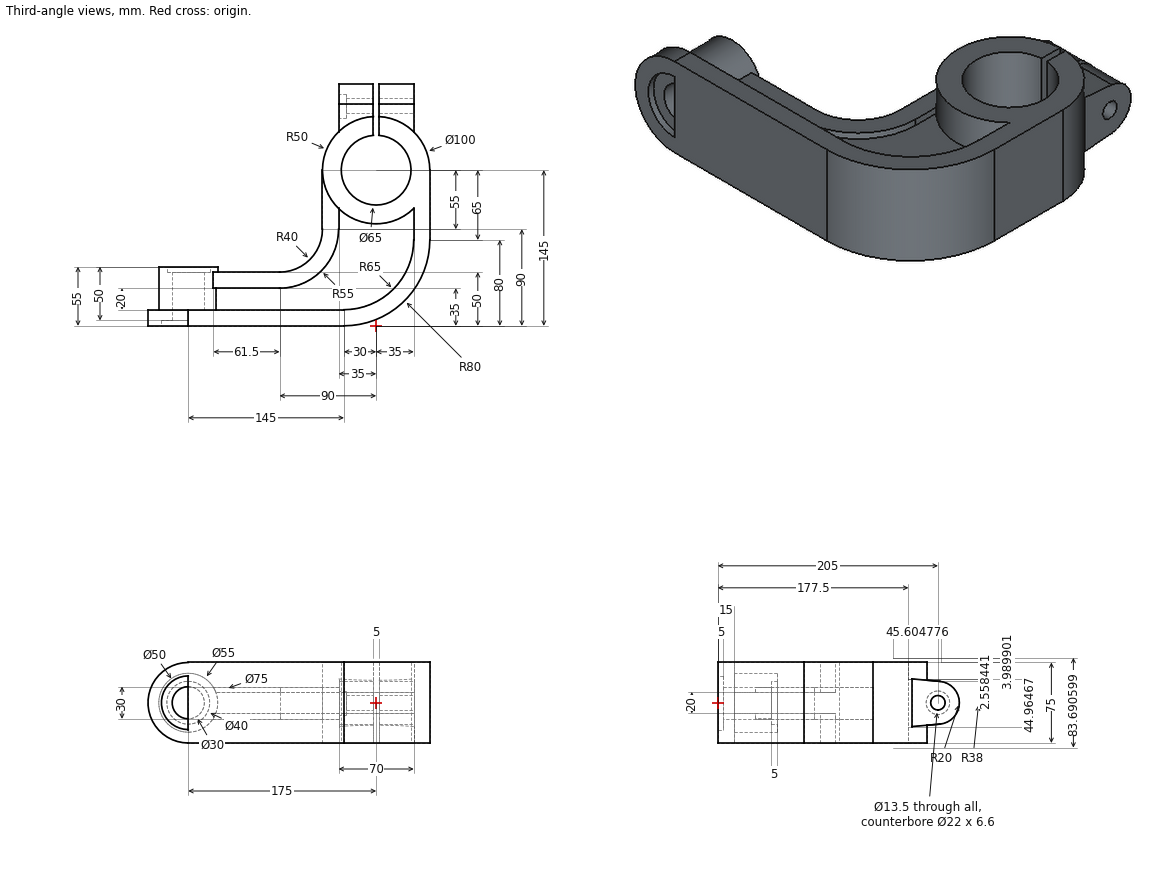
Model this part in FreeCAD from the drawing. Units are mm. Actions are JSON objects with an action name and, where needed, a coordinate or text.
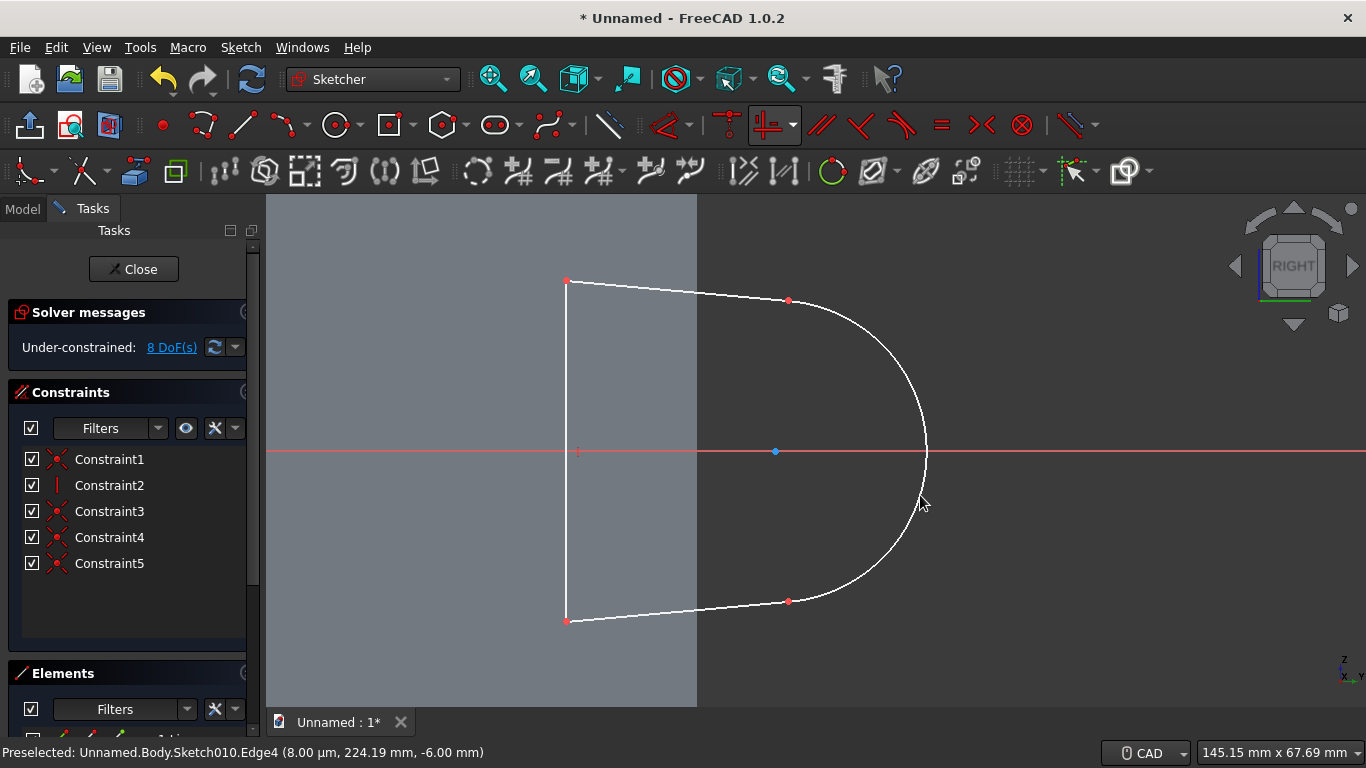
{"action": "left_click", "coordinate": [721, 295]}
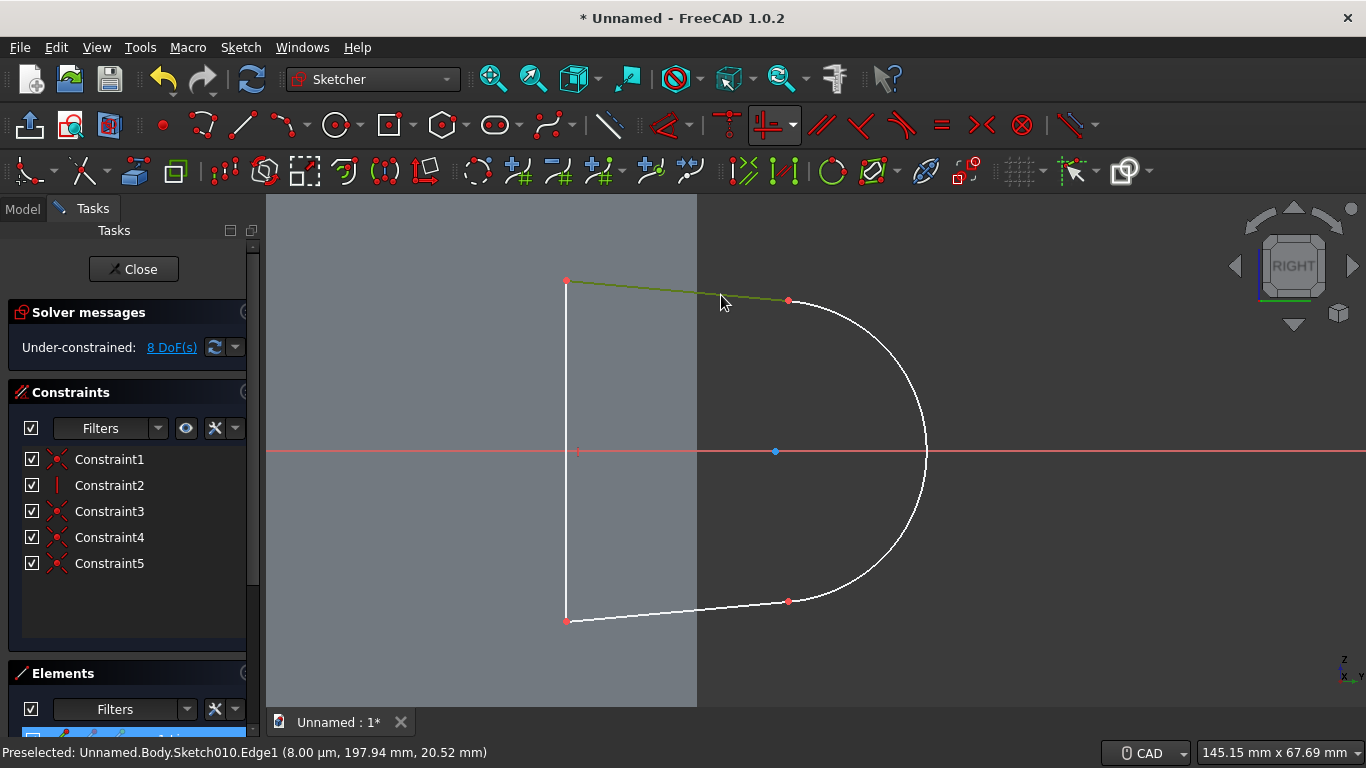
{"action": "left_click", "coordinate": [901, 536]}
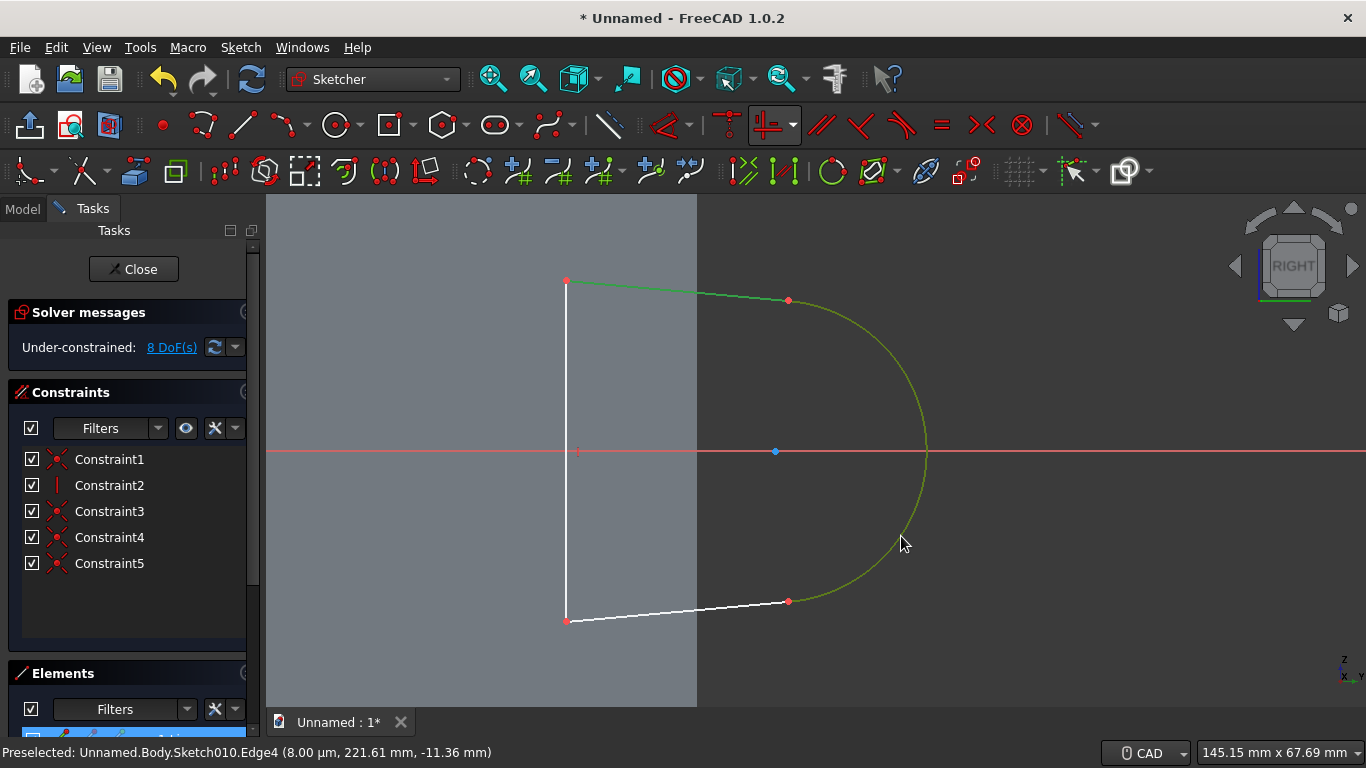
{"action": "key", "text": "t"}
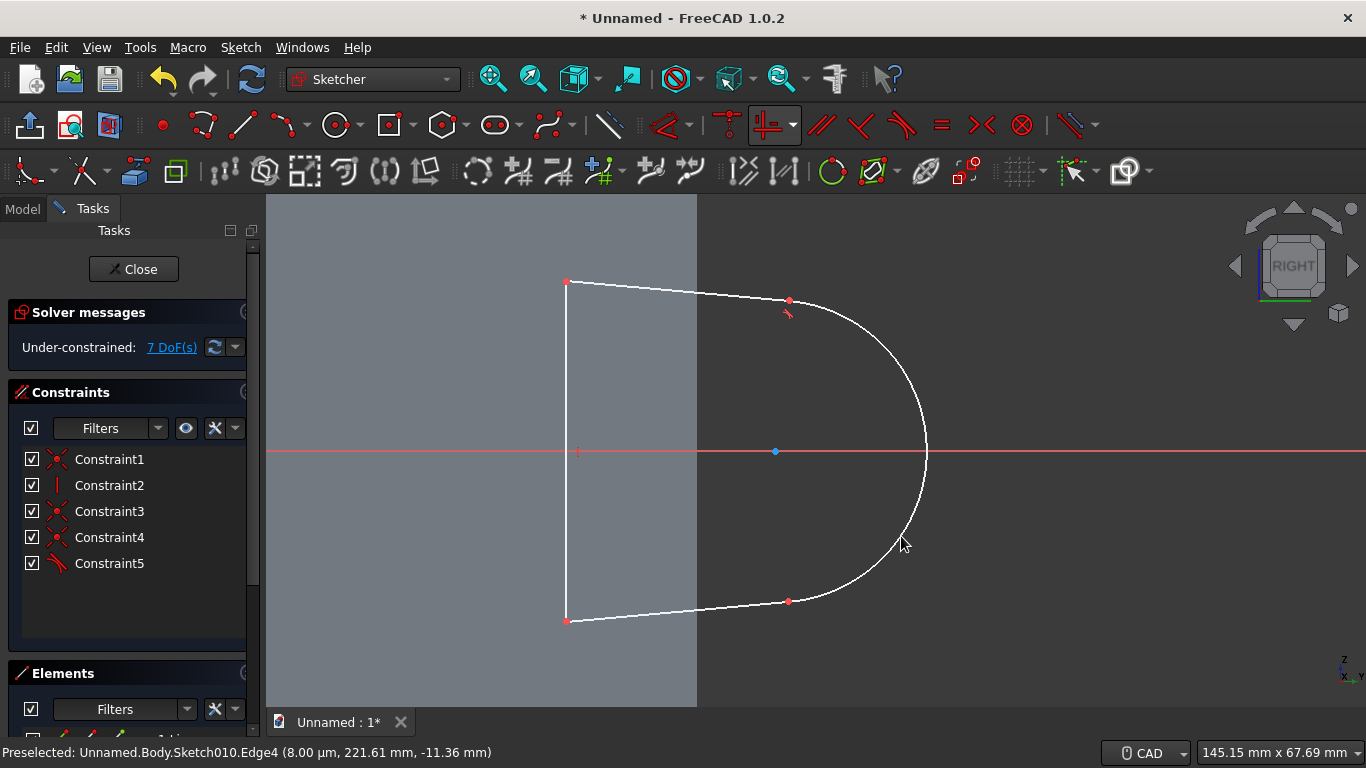
{"action": "left_click", "coordinate": [633, 616]}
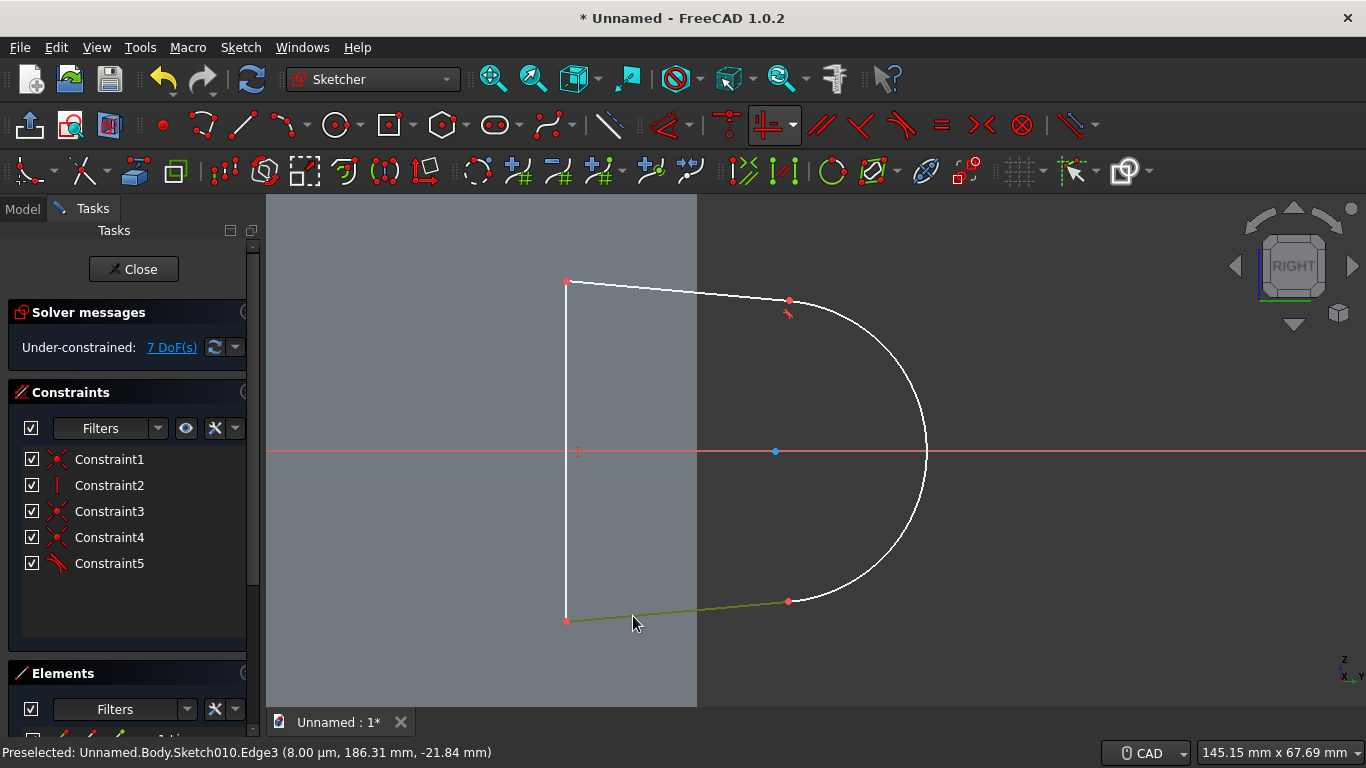
{"action": "left_click", "coordinate": [901, 537]}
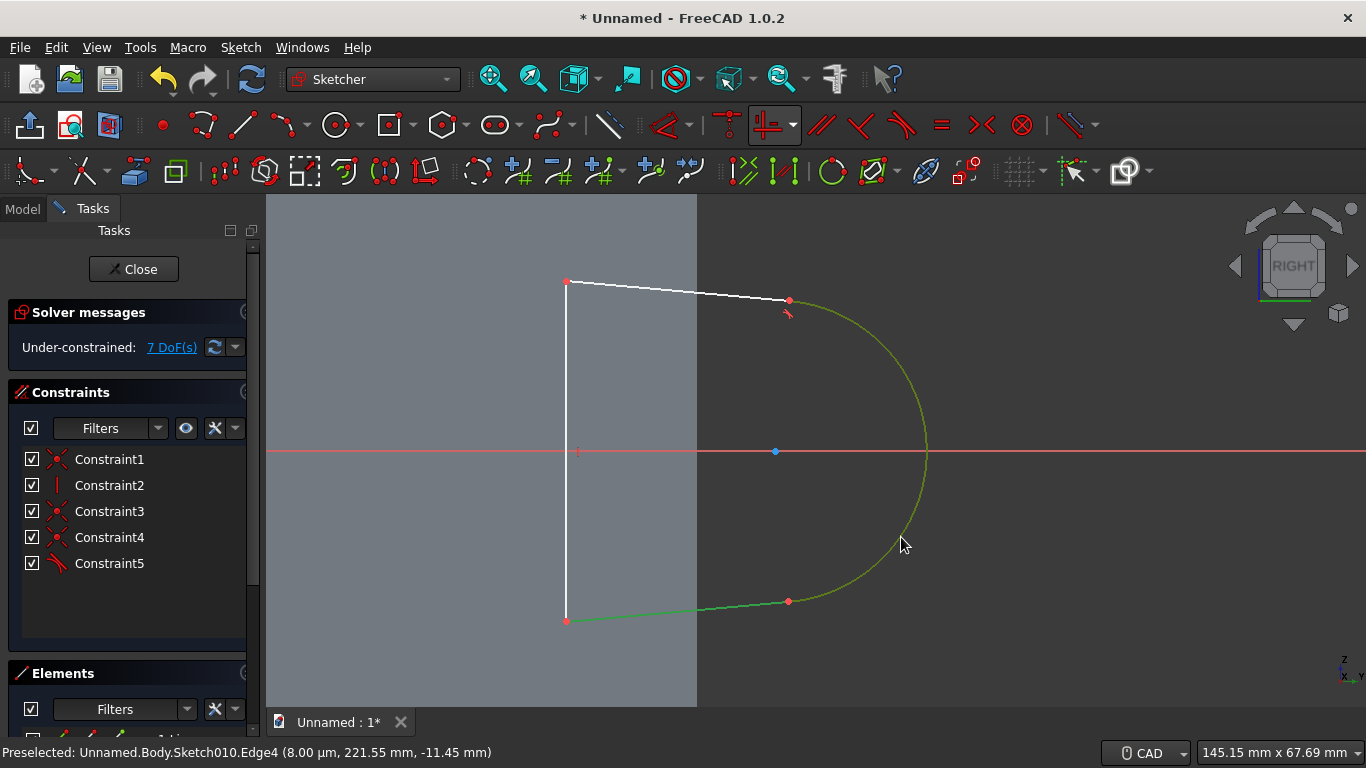
{"action": "key", "text": "t"}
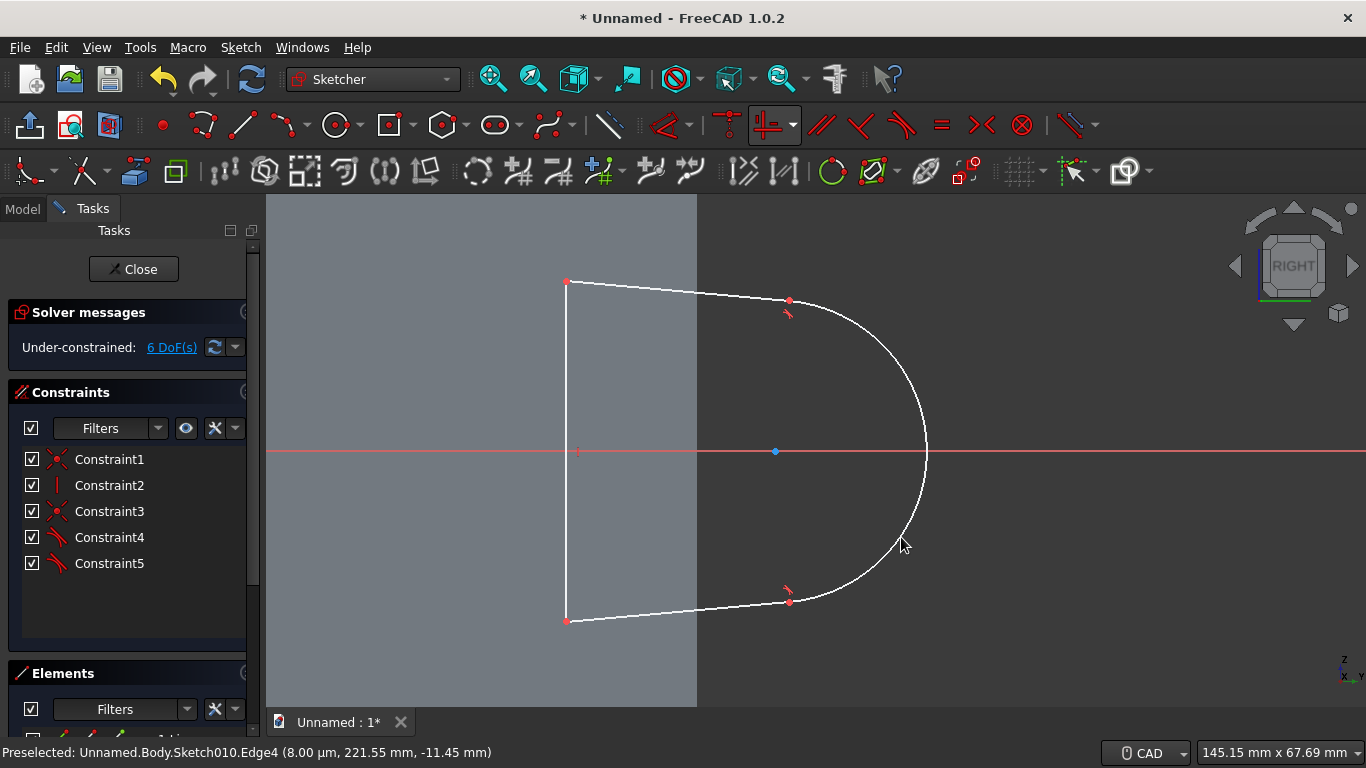
{"action": "left_click", "coordinate": [776, 451]}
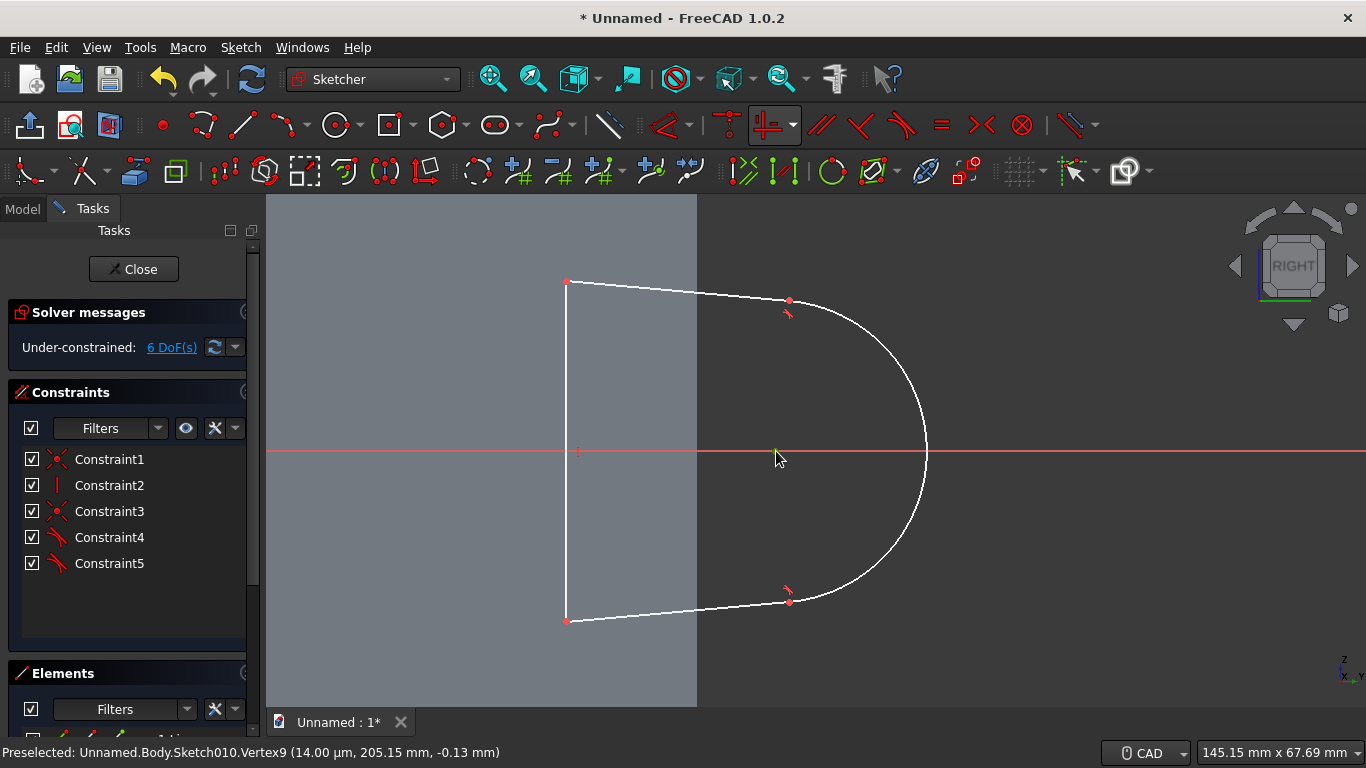
{"action": "left_click", "coordinate": [359, 450]}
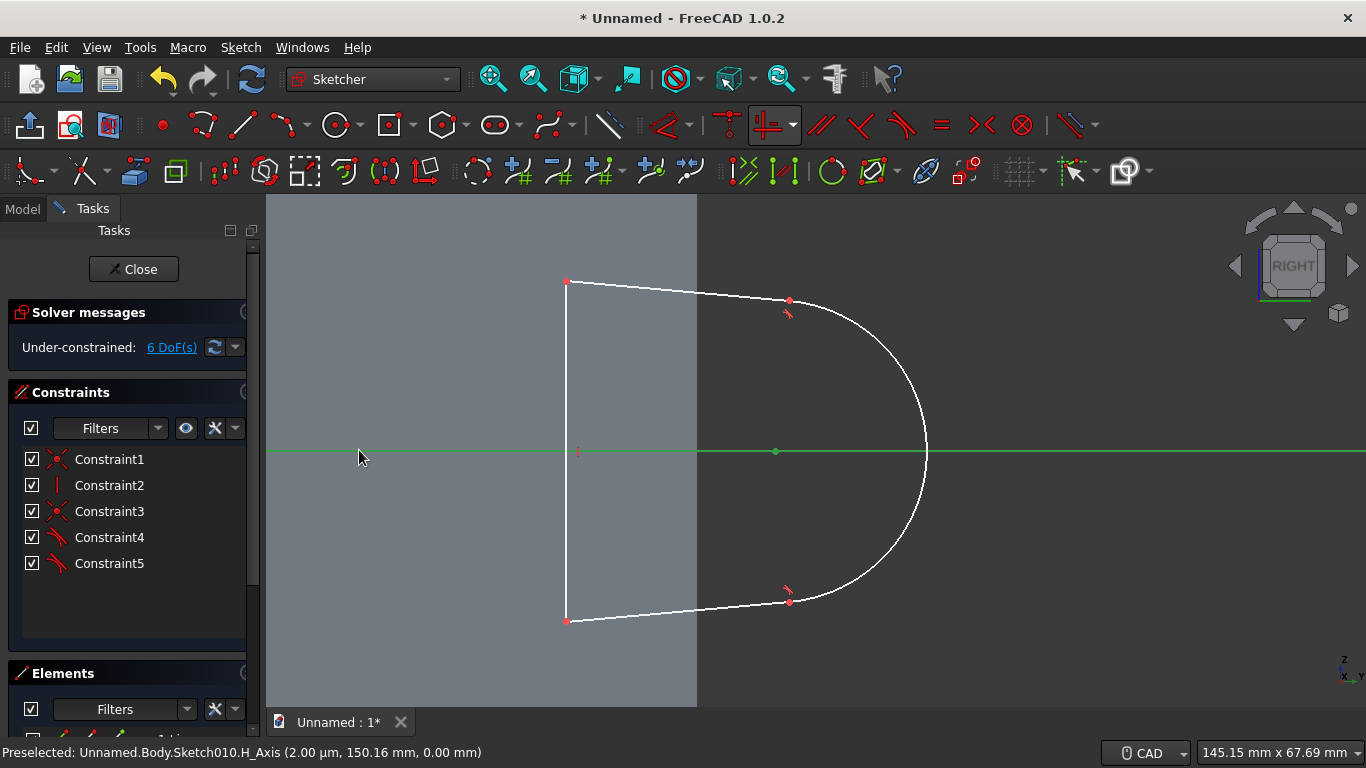
{"action": "key", "text": "c"}